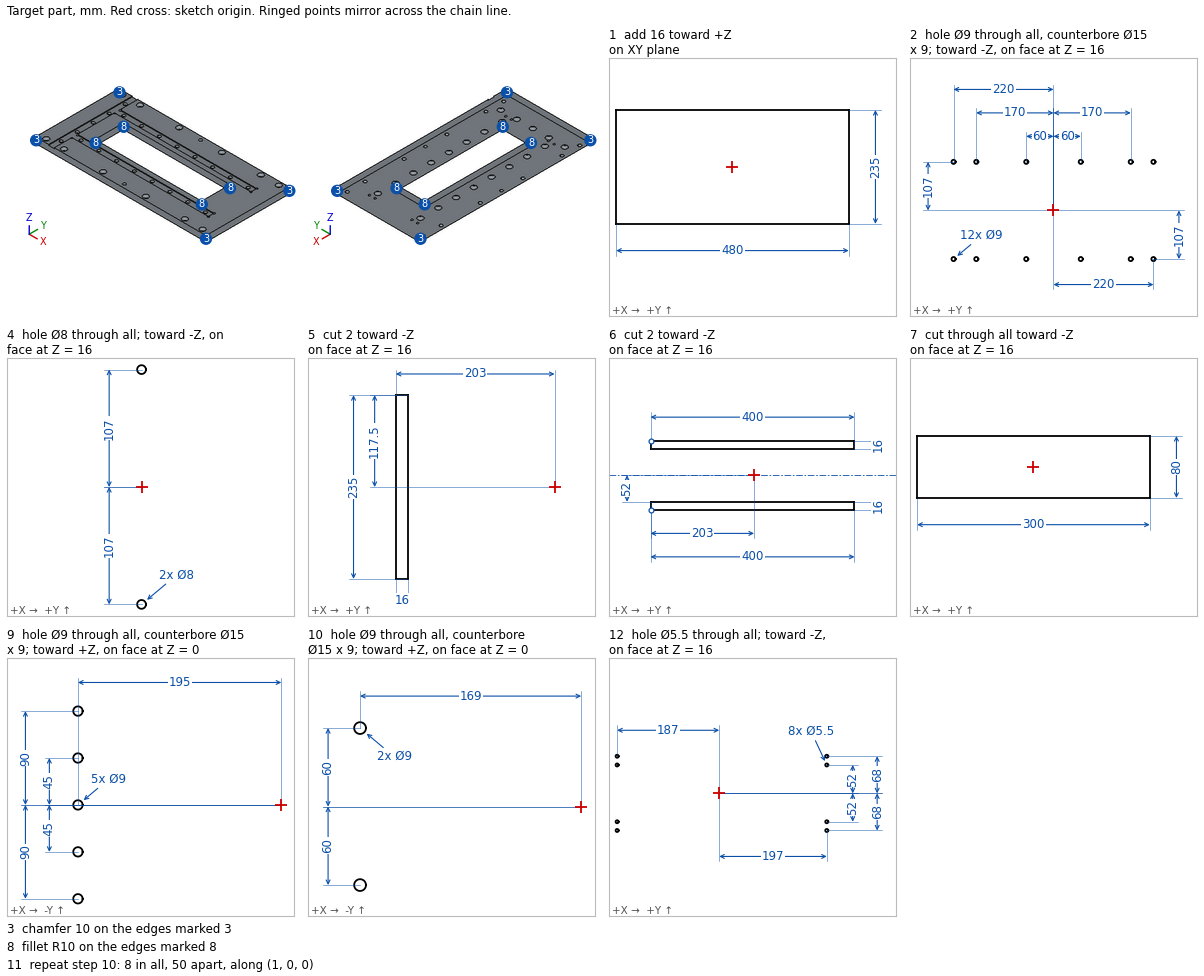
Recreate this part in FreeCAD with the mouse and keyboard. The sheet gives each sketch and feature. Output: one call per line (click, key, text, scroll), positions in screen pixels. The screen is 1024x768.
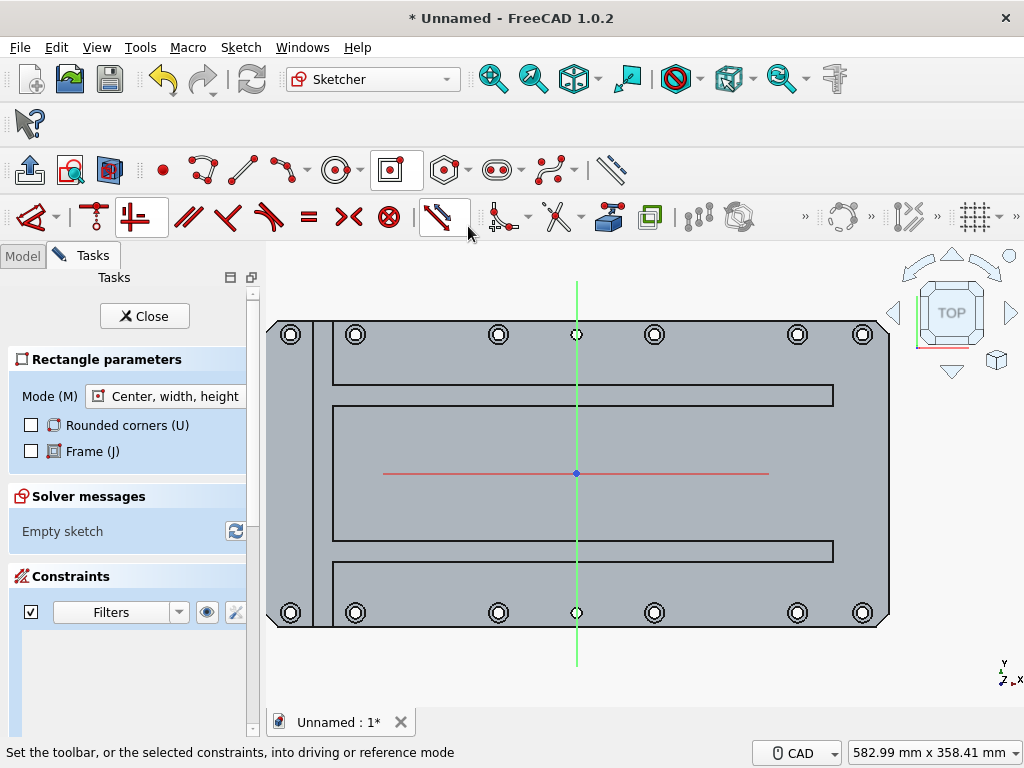
click(577, 474)
move(772, 422)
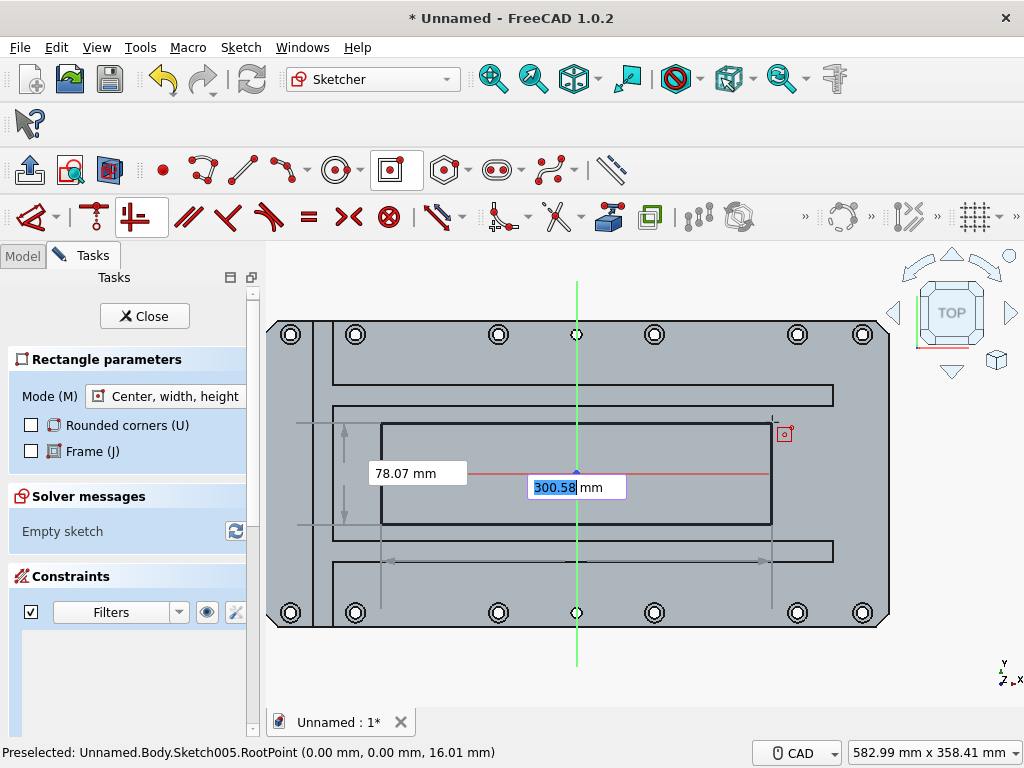
text(300)
key(Tab)
text(80)
key(Return)
key(Escape)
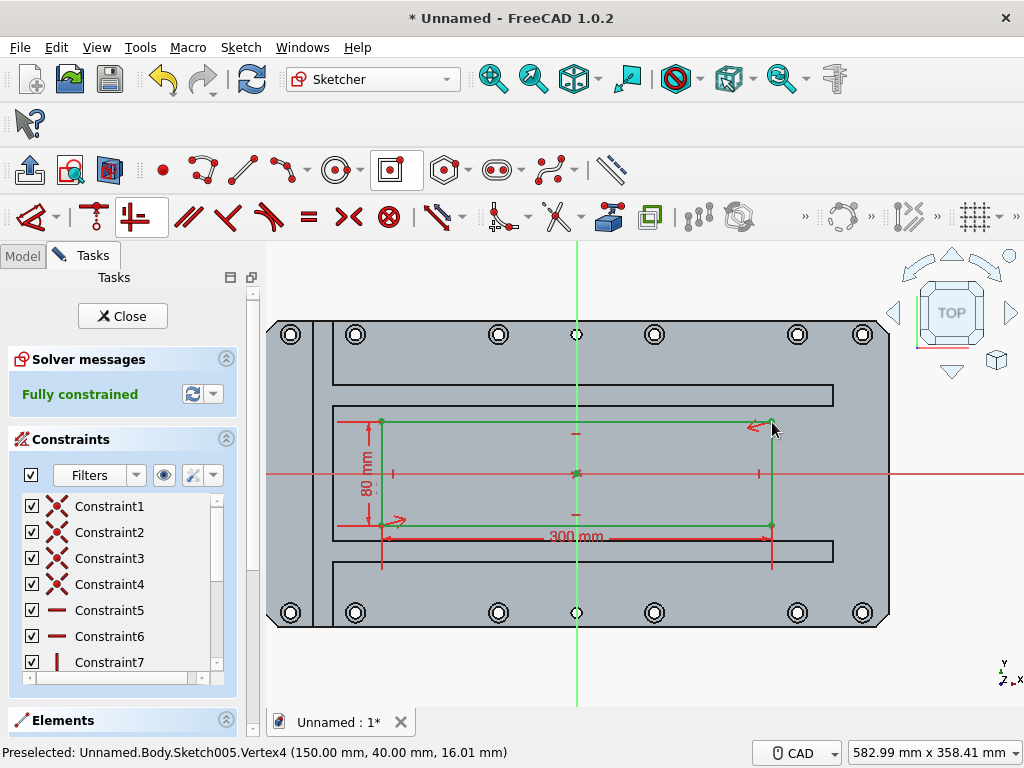
click(123, 316)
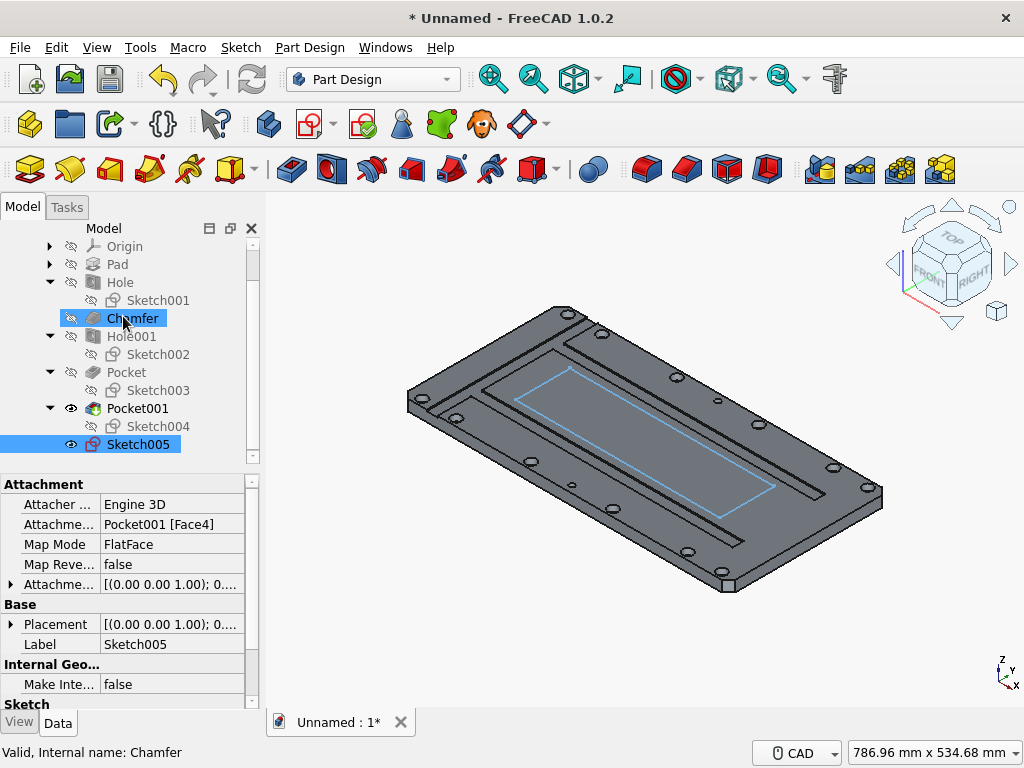
click(292, 170)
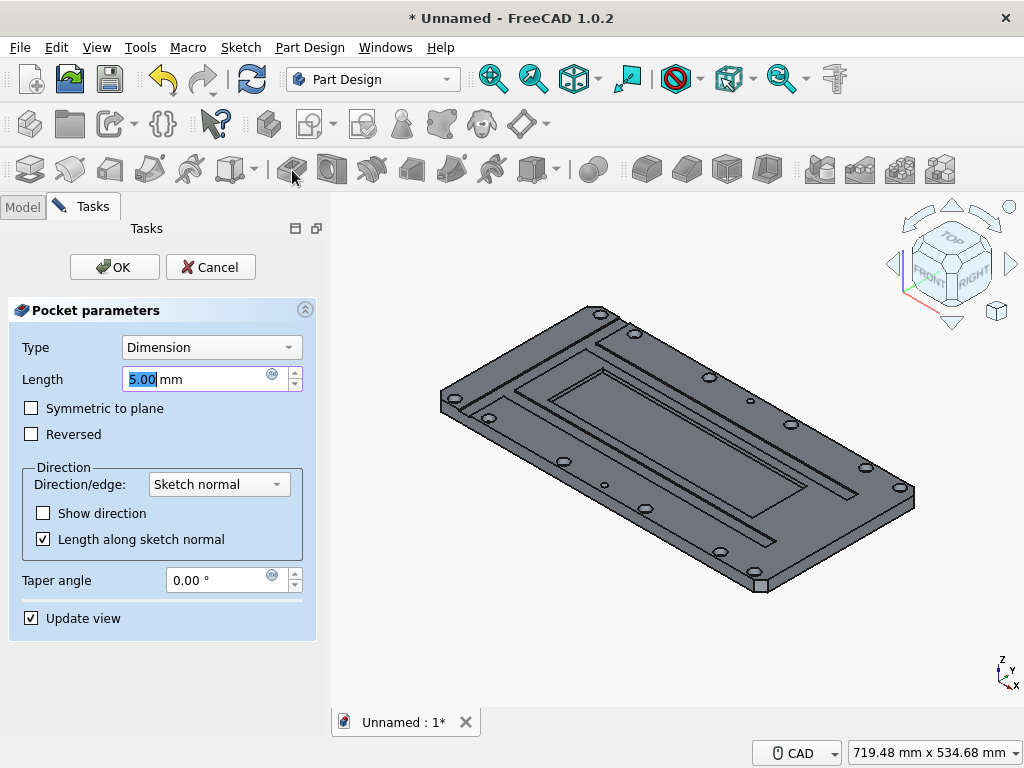
click(212, 348)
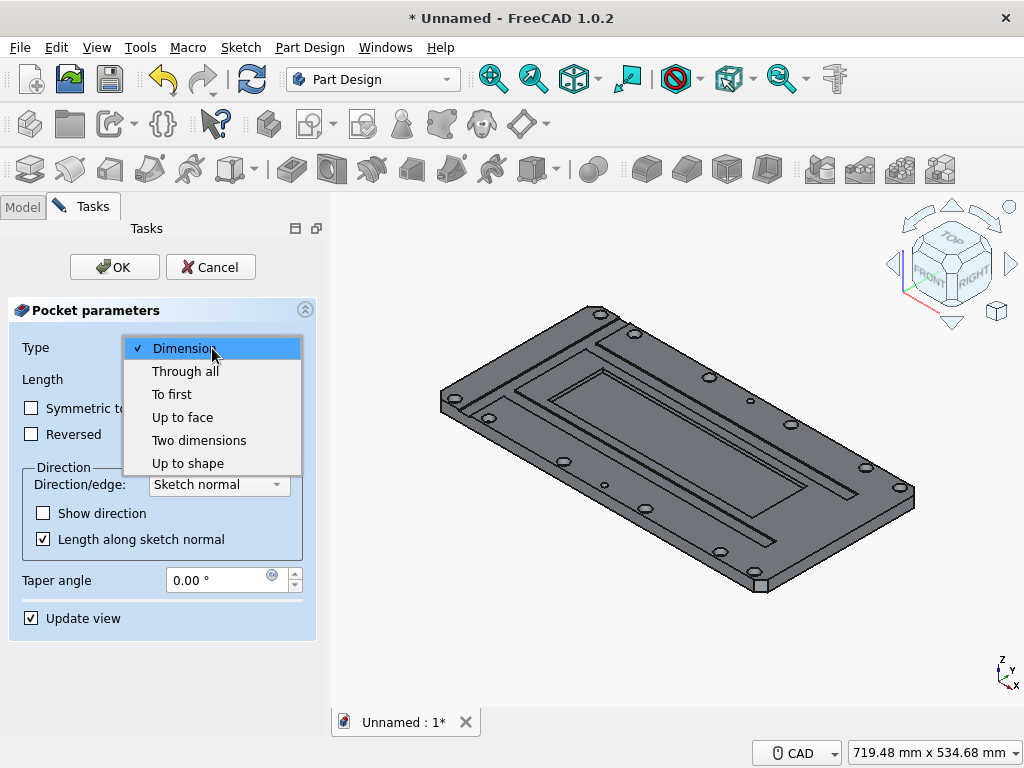
click(212, 372)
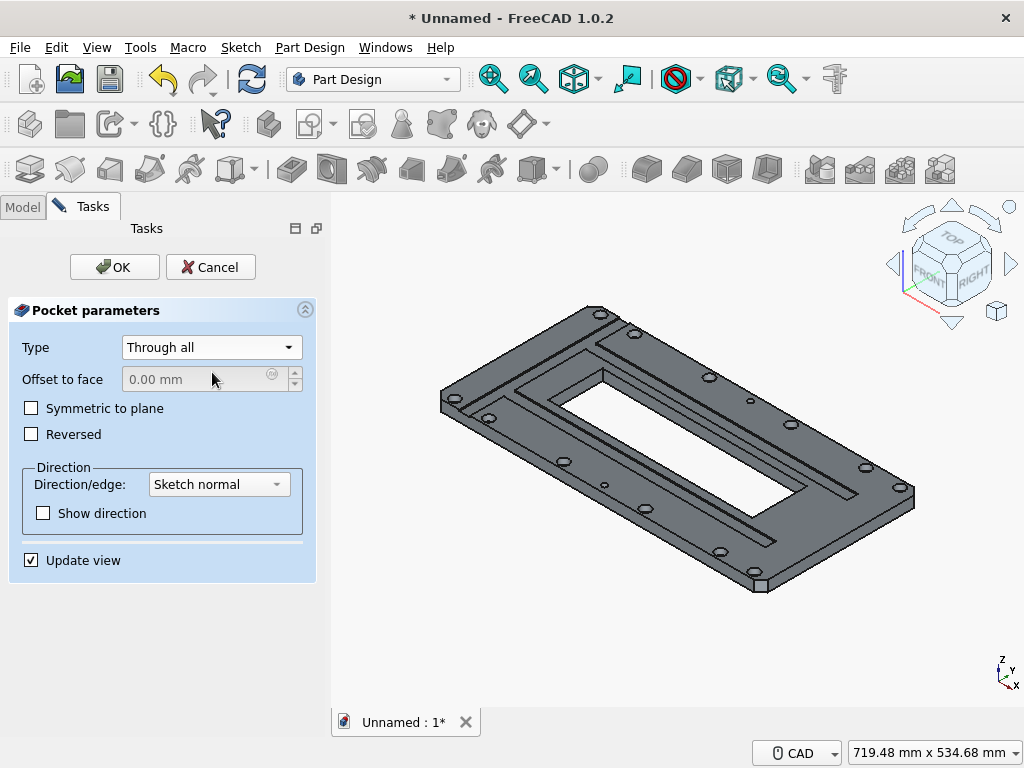
click(115, 267)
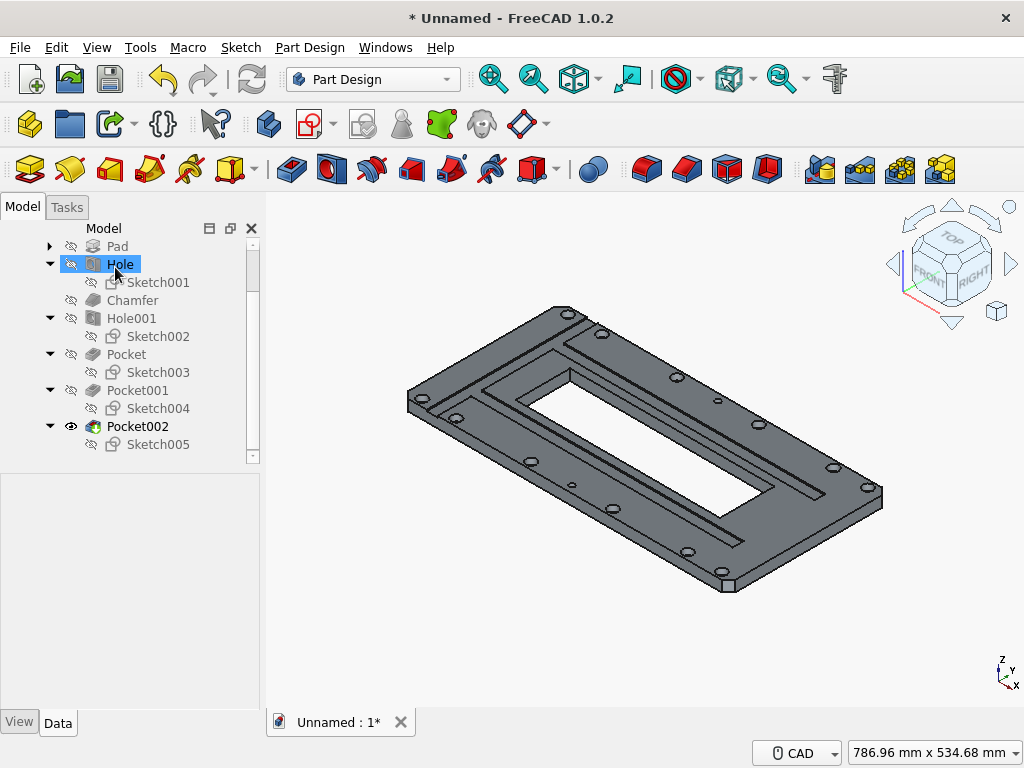
scroll(774, 492, up, 5)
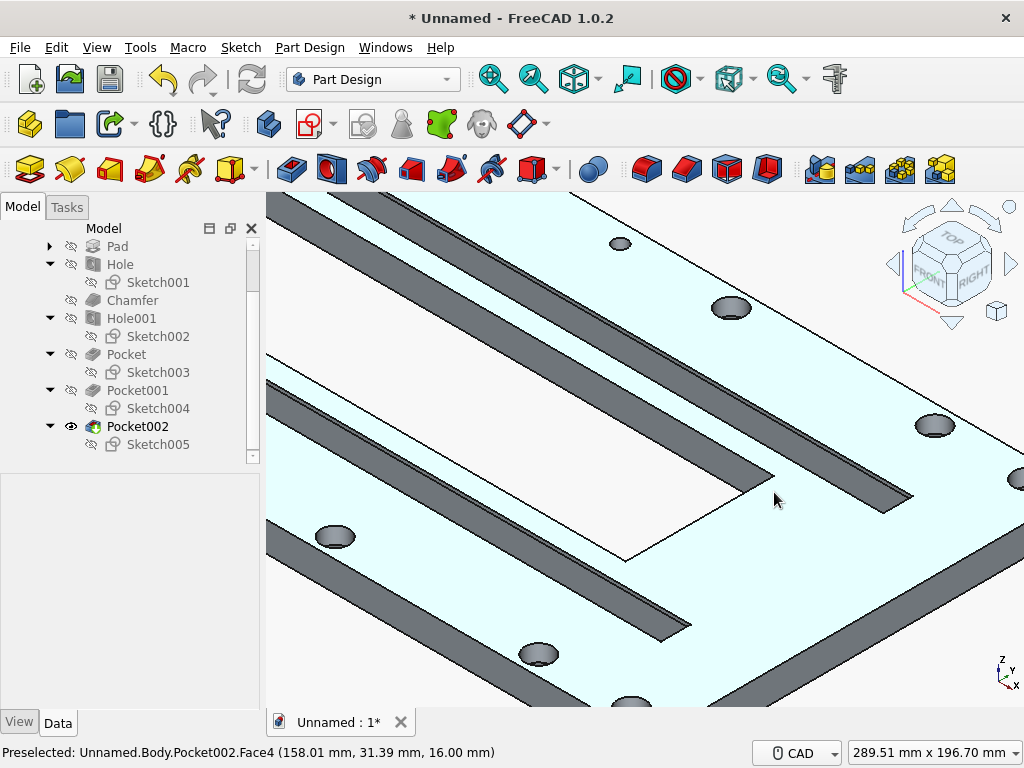
click(494, 80)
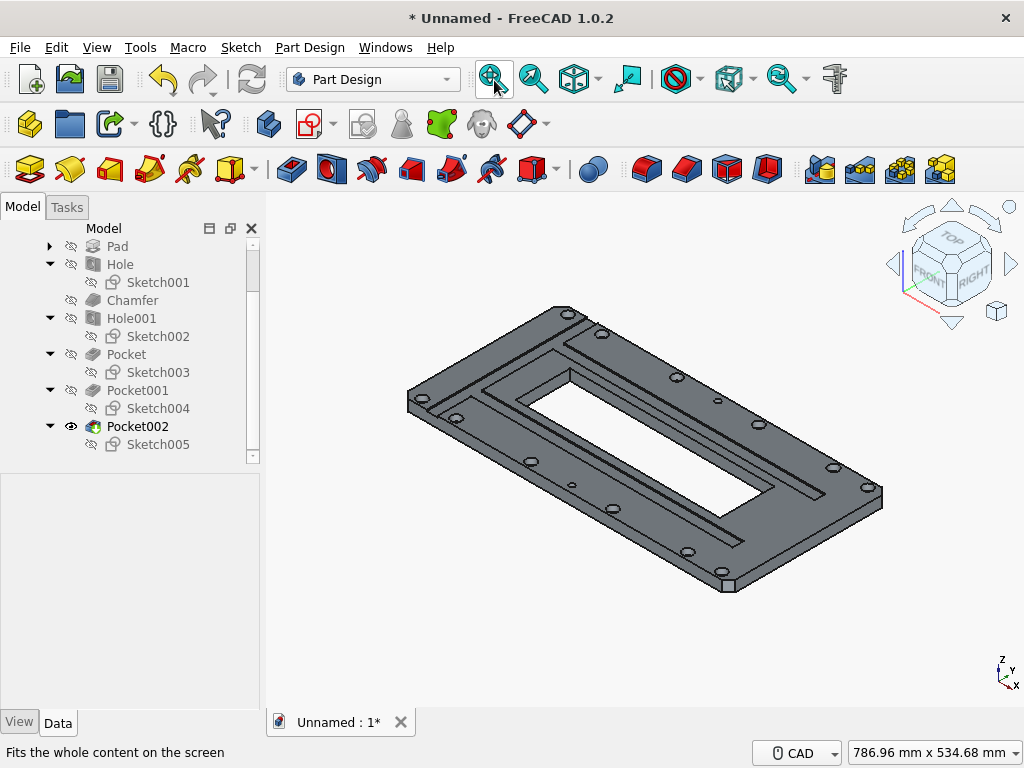
key(2)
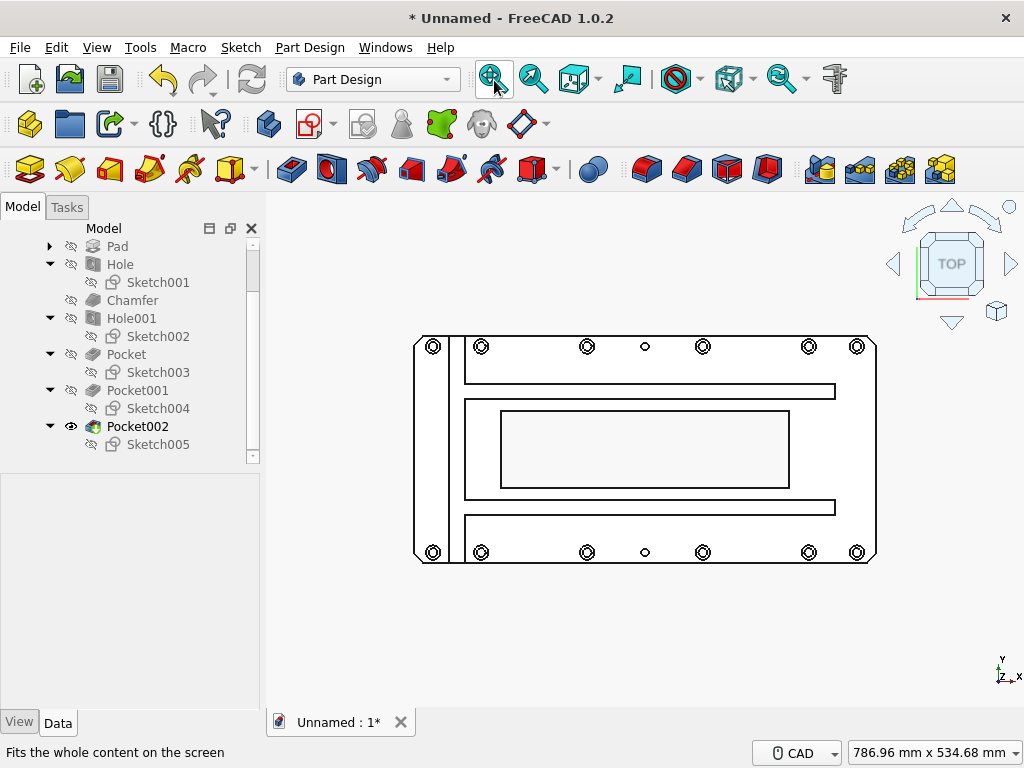
scroll(789, 410, up, 5)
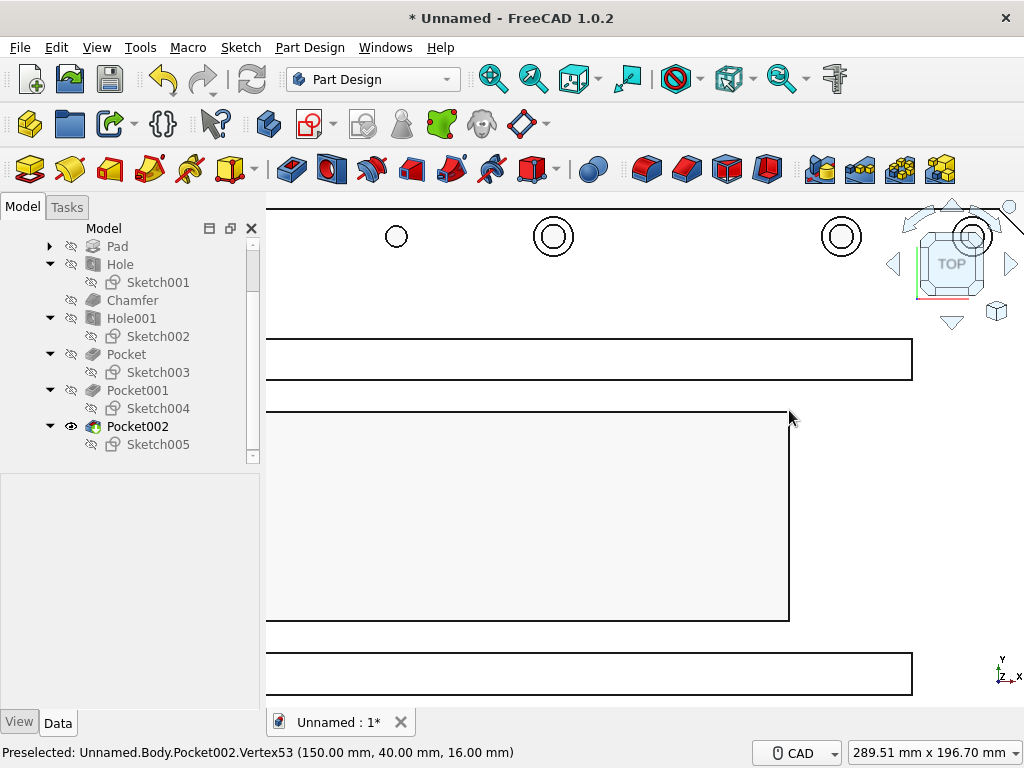
click(494, 80)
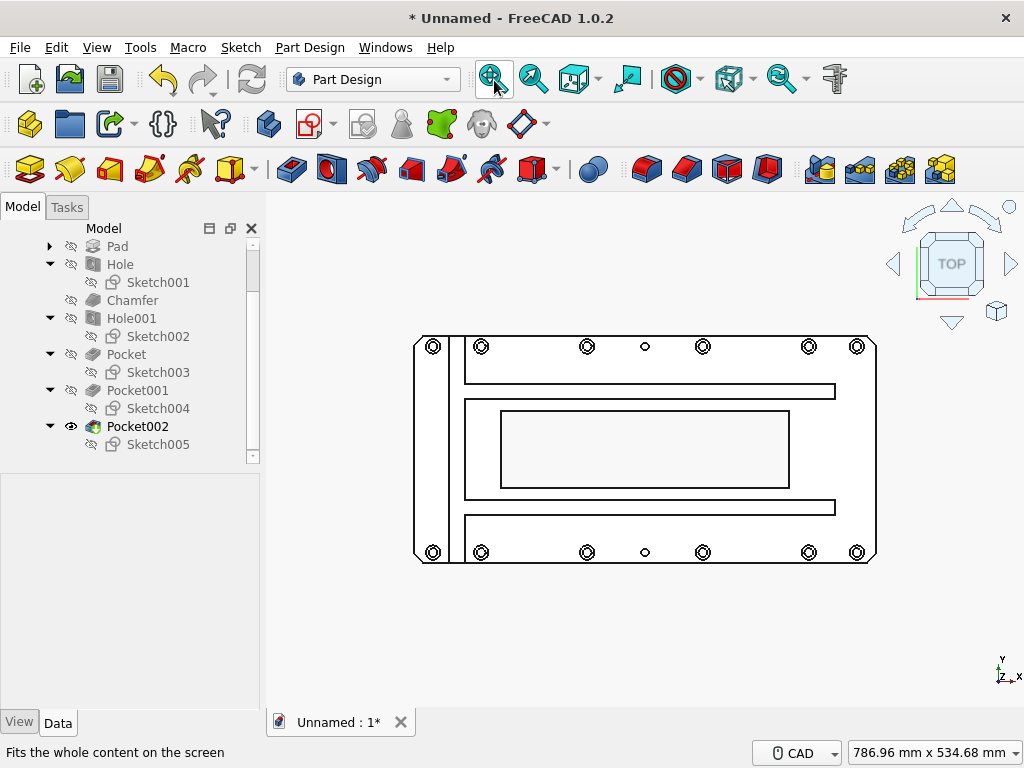
key(0)